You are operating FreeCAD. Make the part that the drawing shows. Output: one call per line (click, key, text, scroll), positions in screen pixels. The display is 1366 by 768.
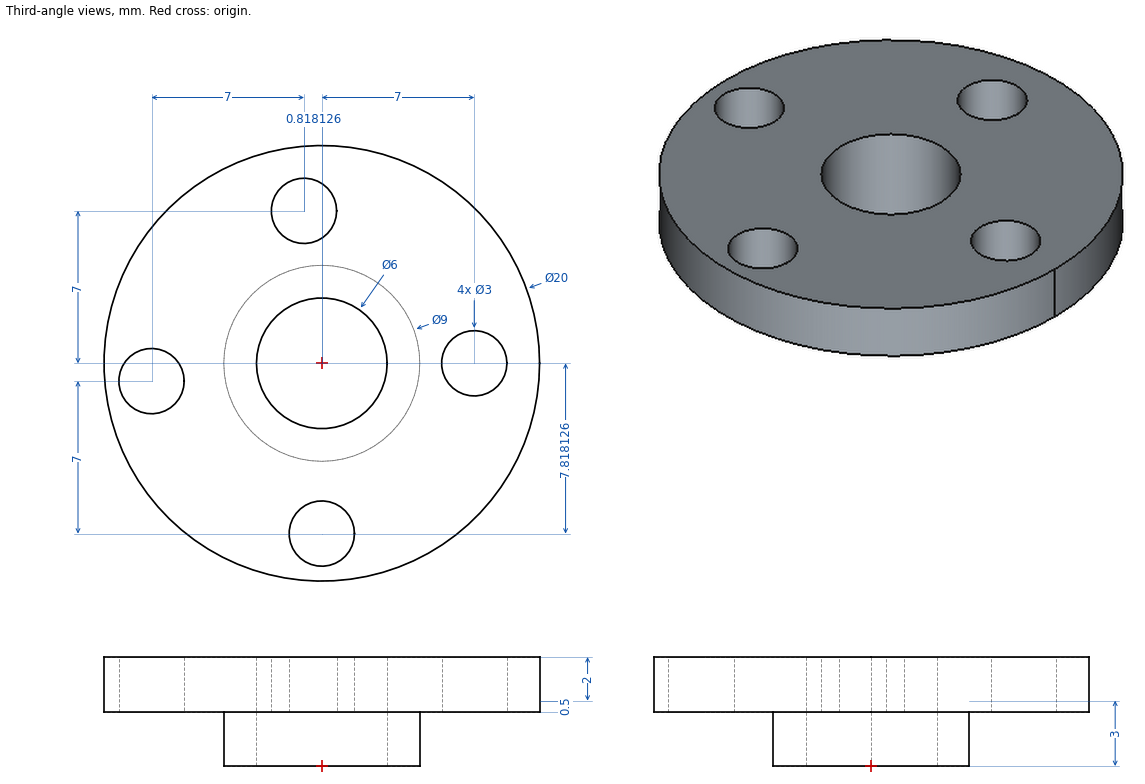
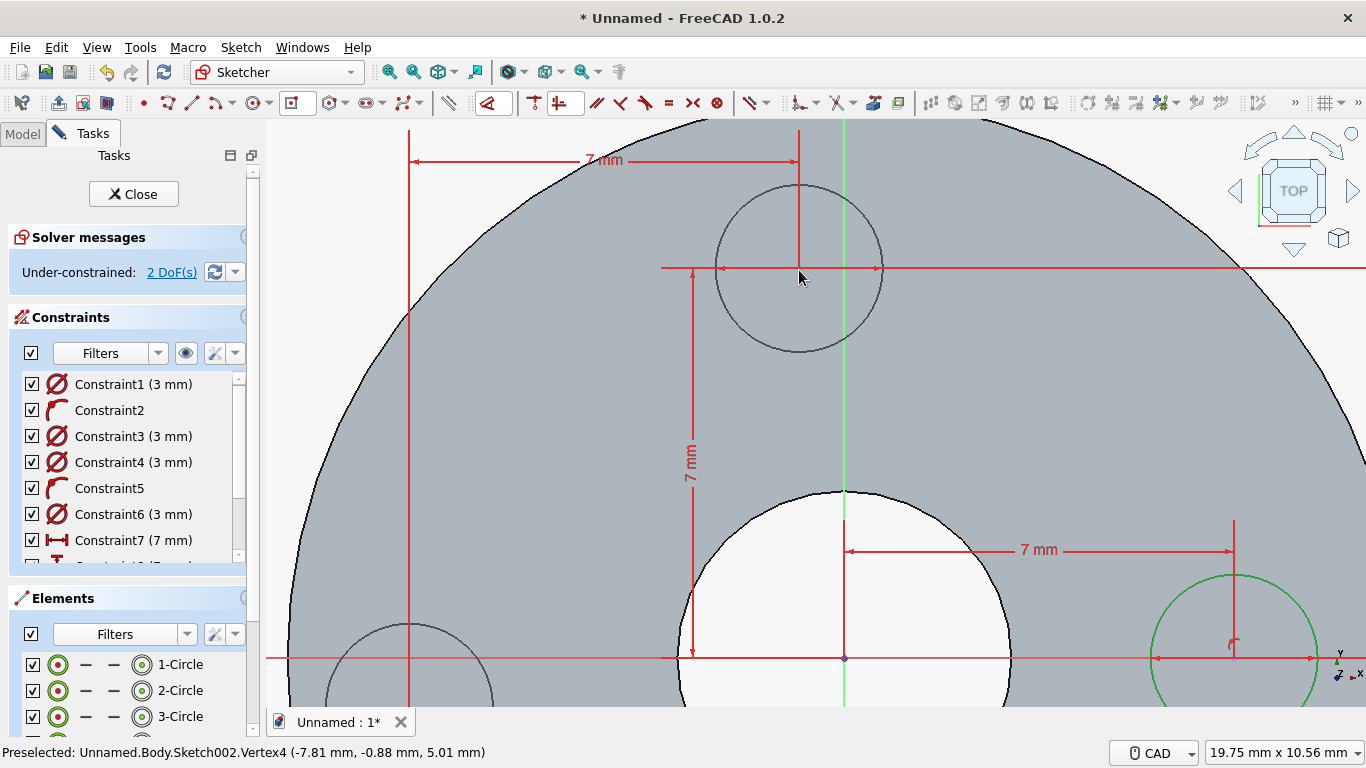
click(799, 268)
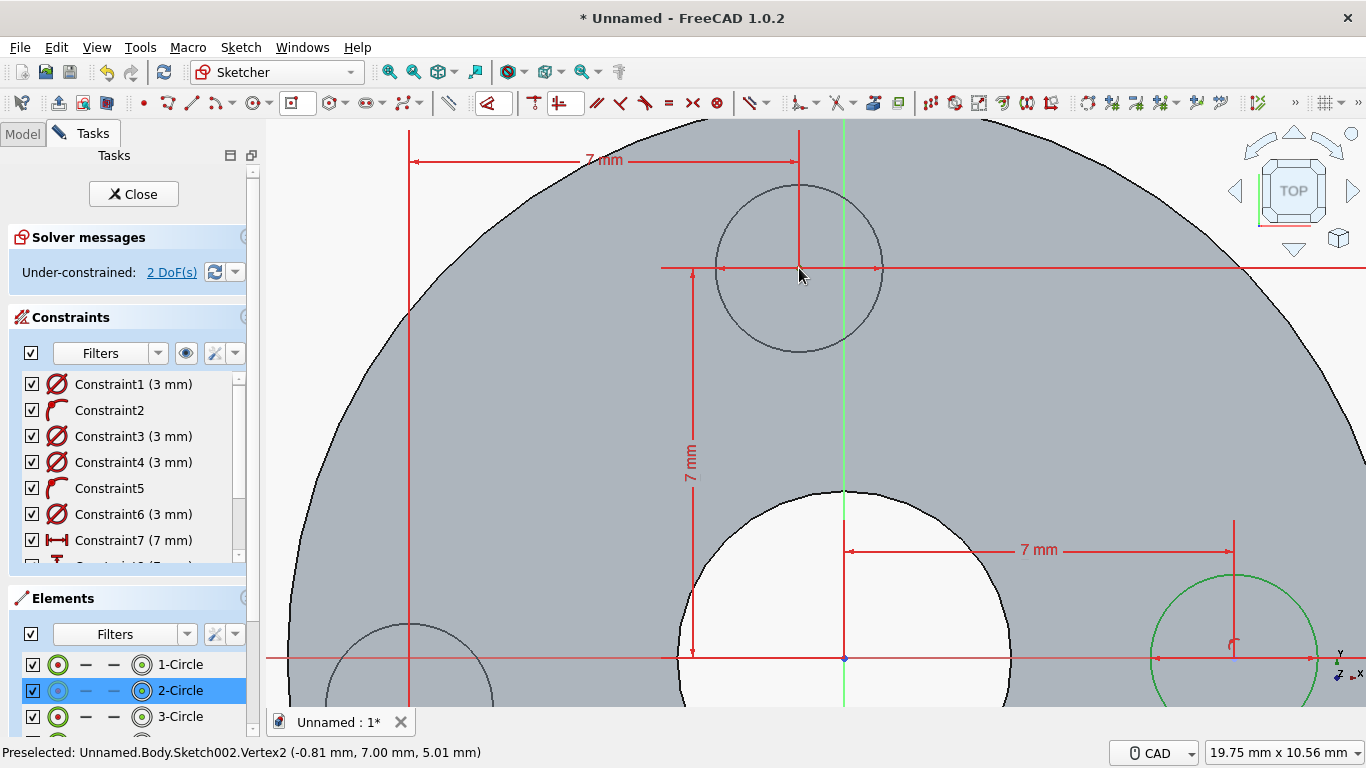
key(l)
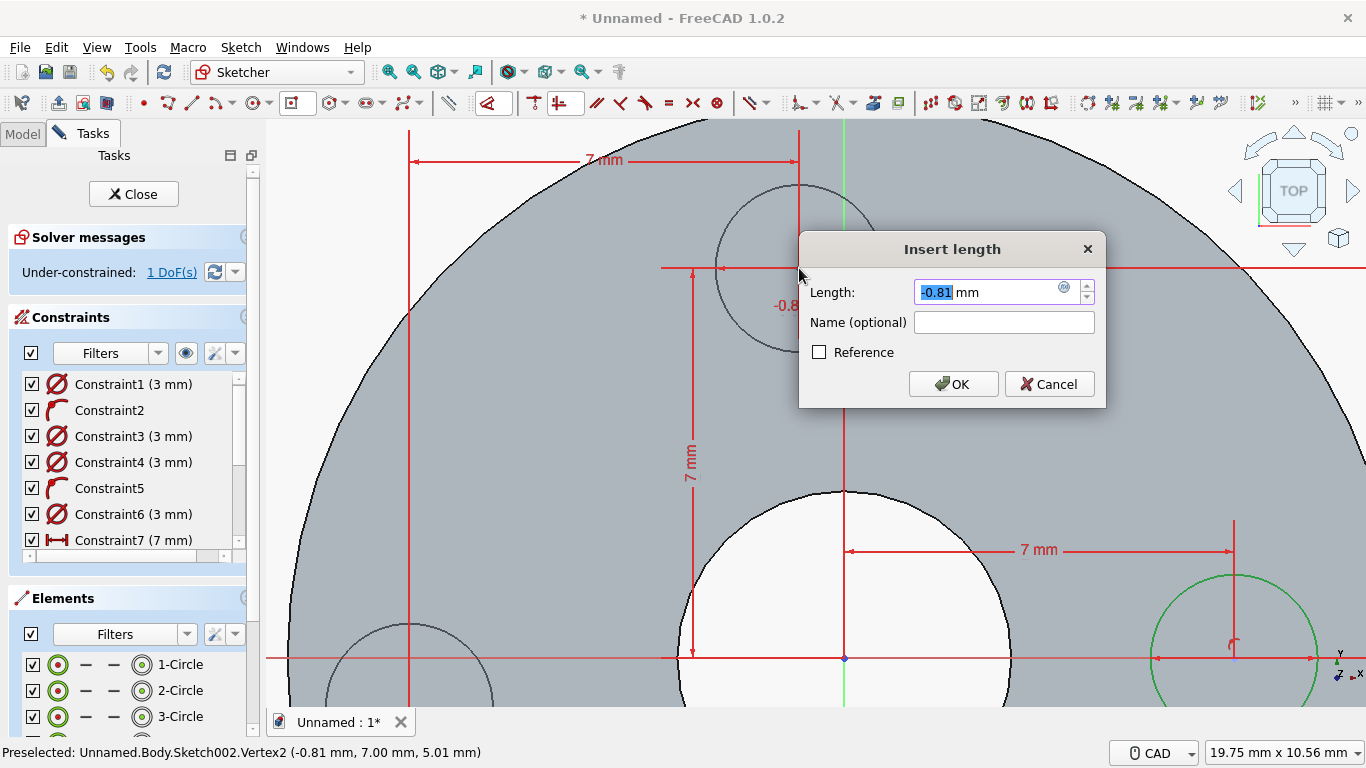
text(-0.818126)
key(Return)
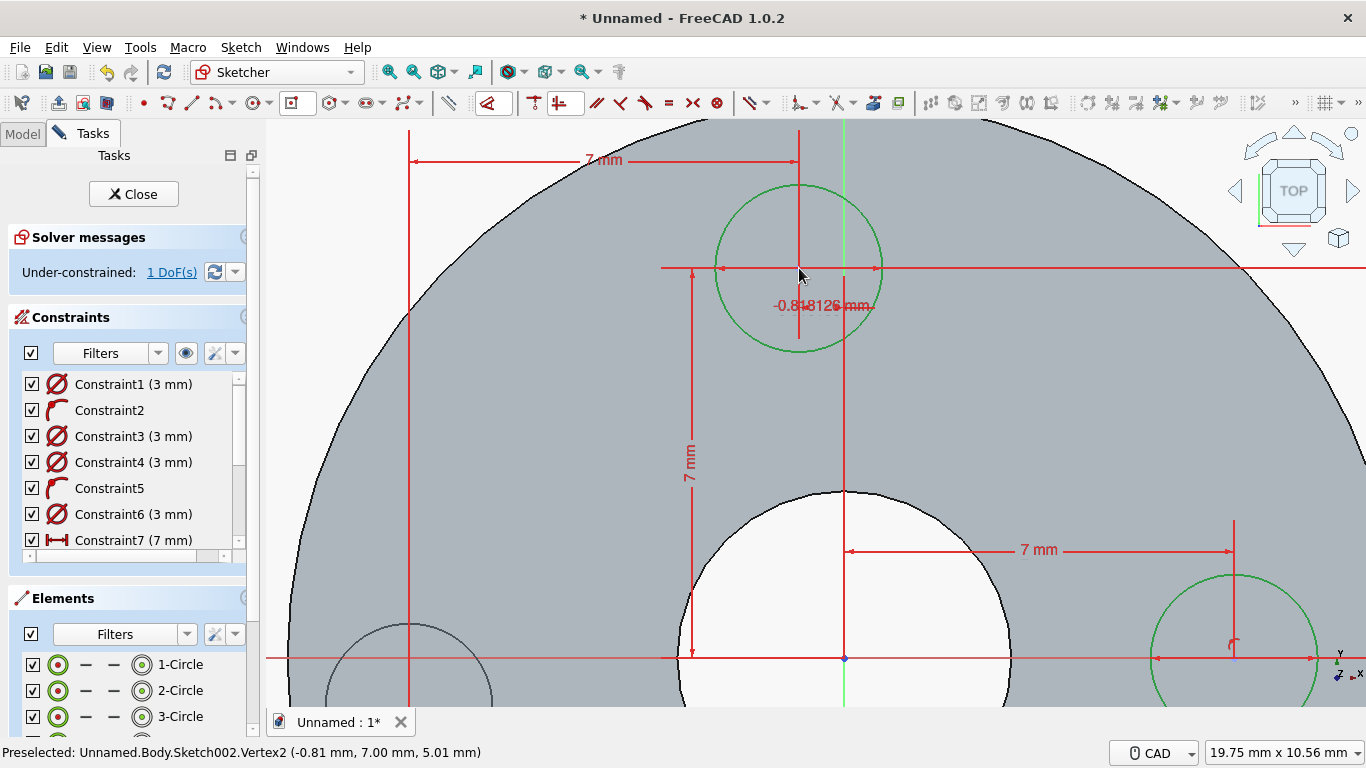
scroll(704, 257, down, 5)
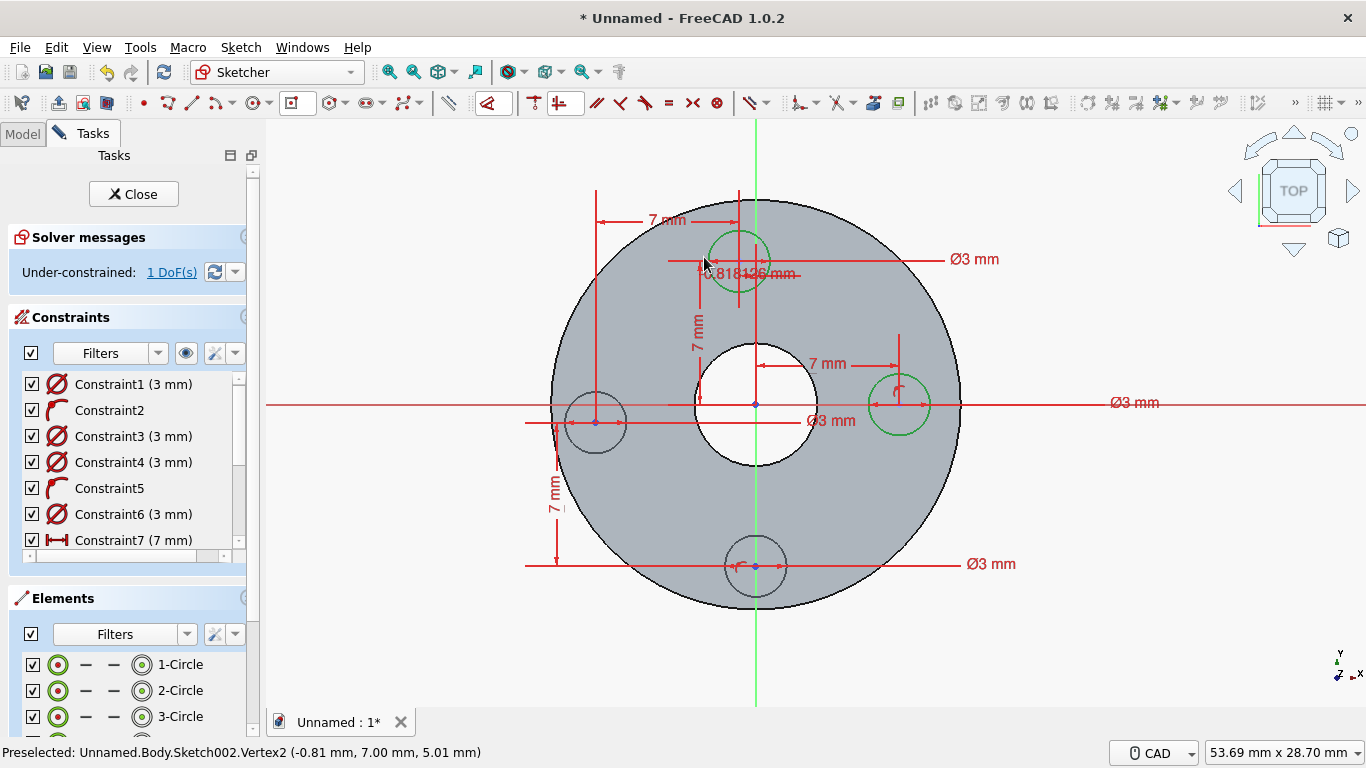
click(756, 566)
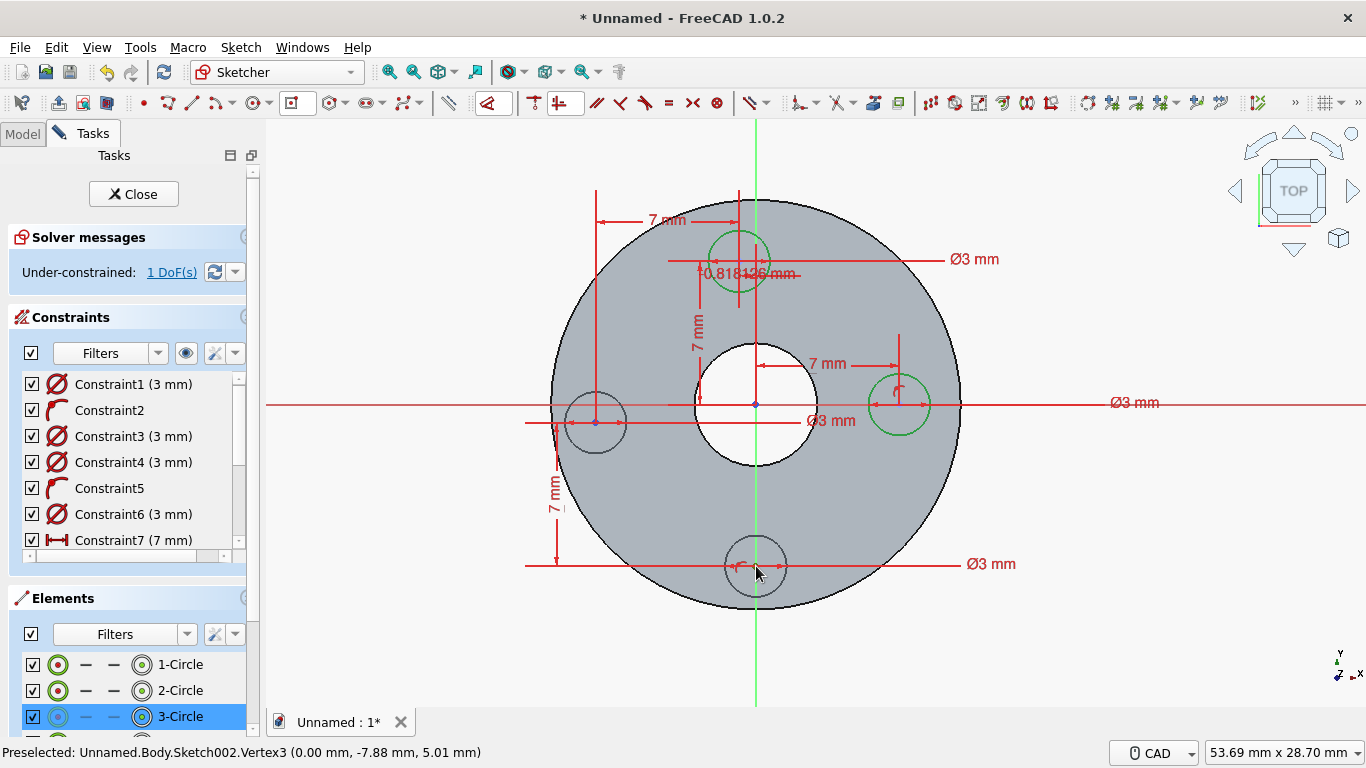
key(i)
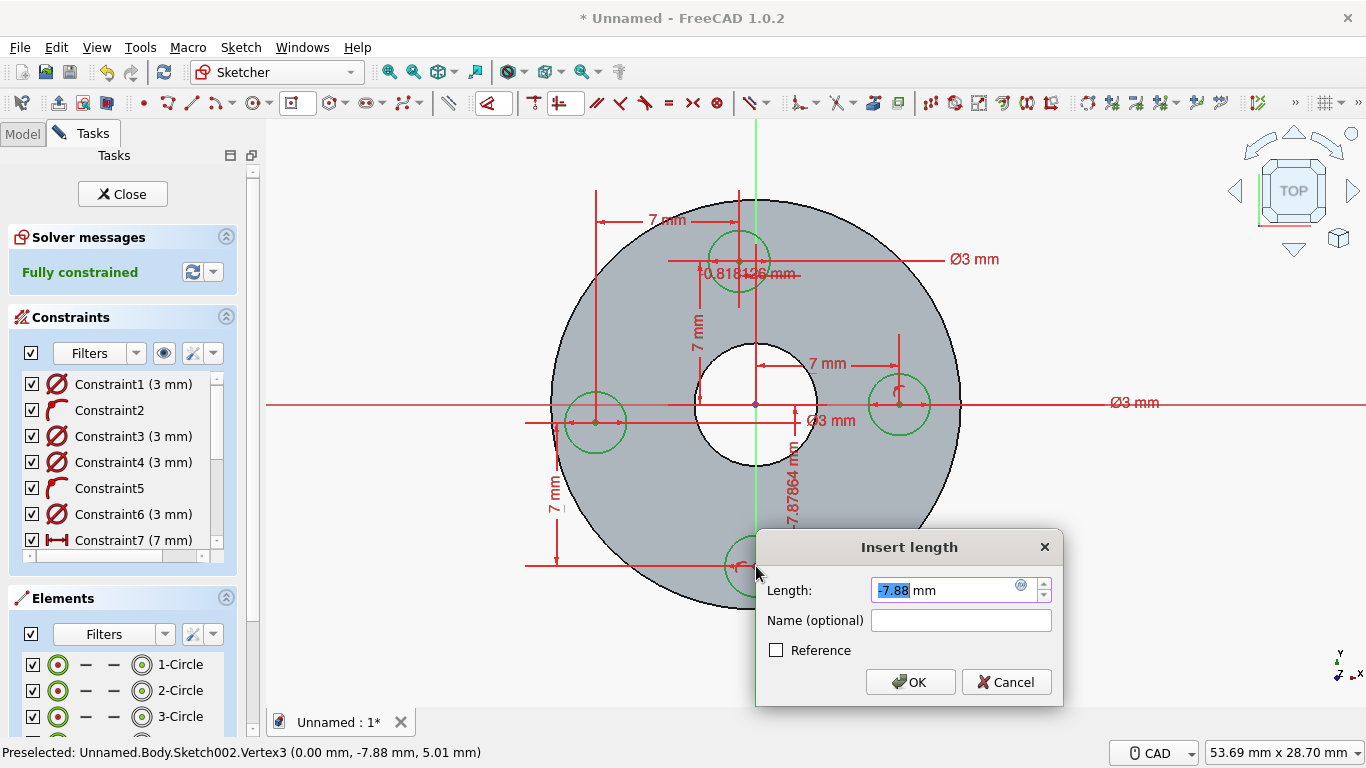
text(-7.818126)
key(Return)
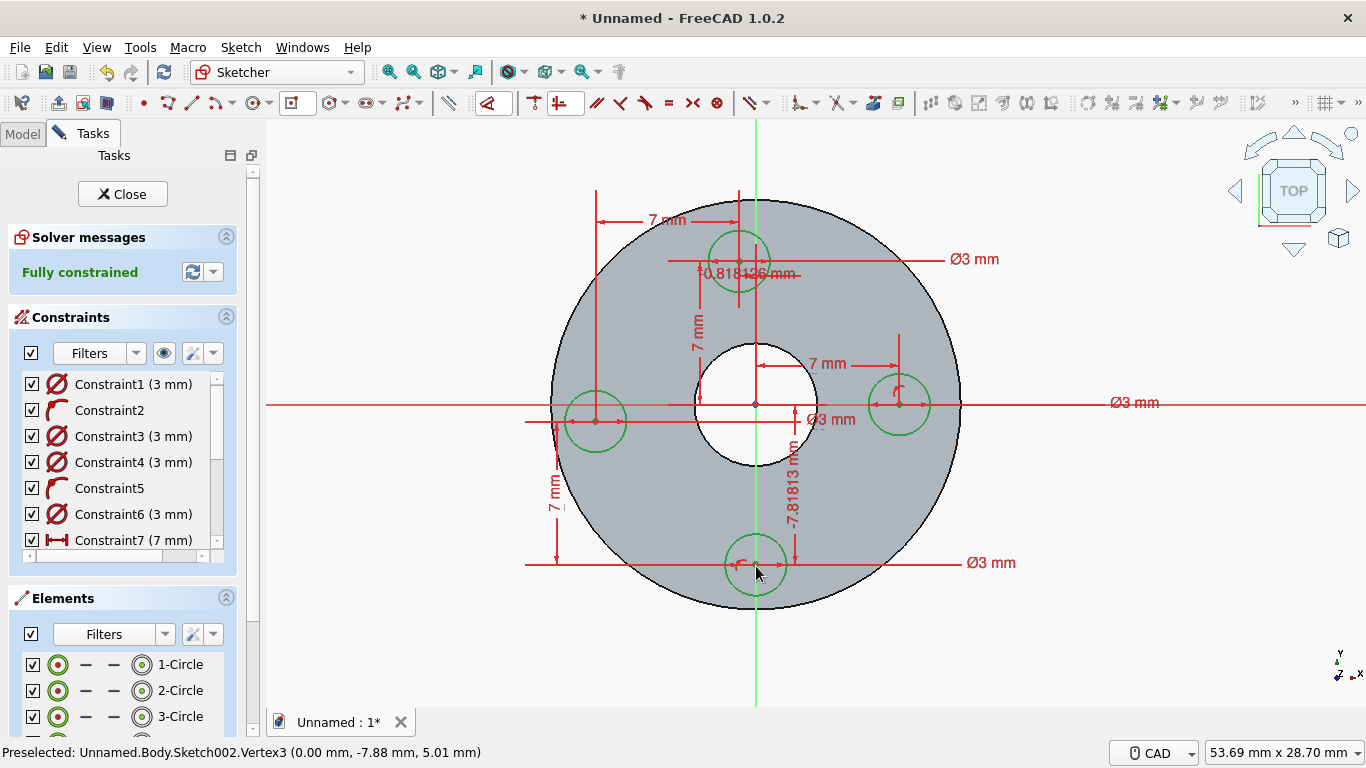
click(123, 194)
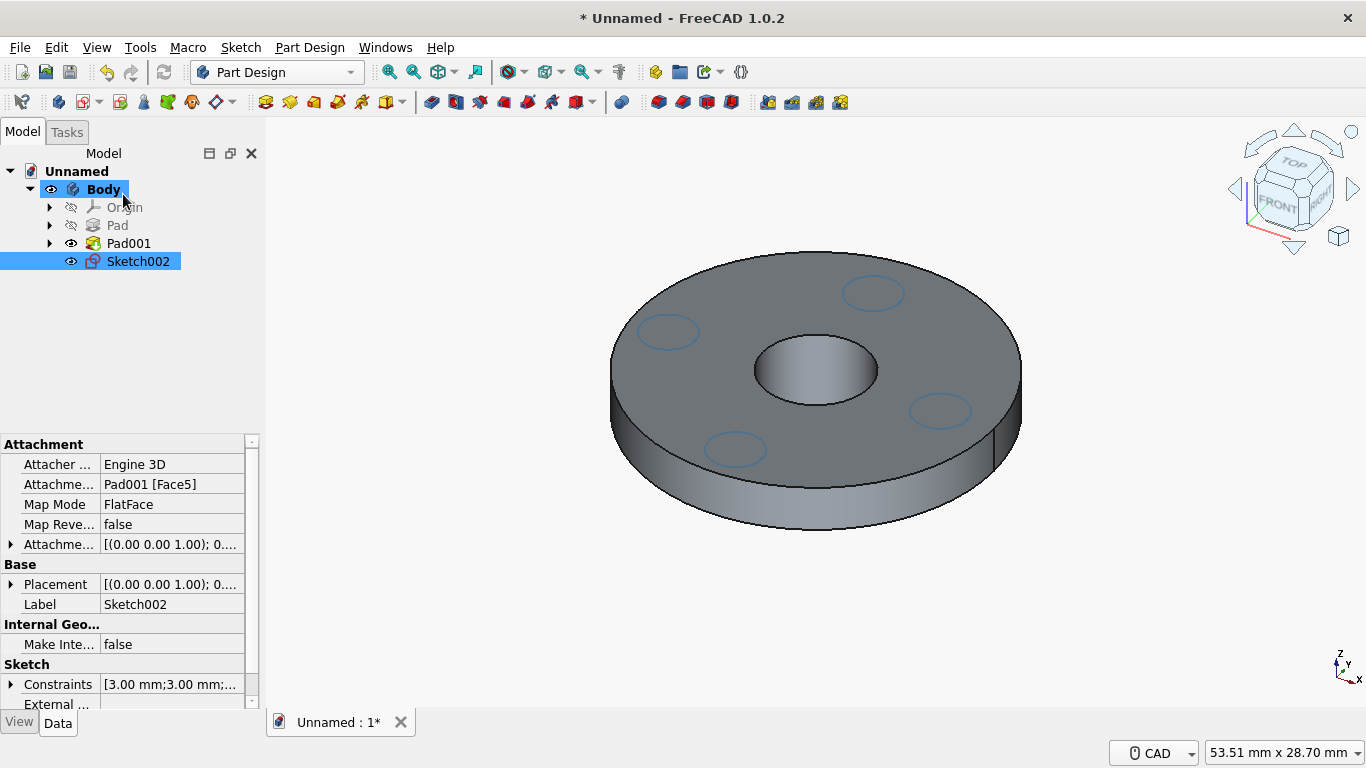
click(432, 102)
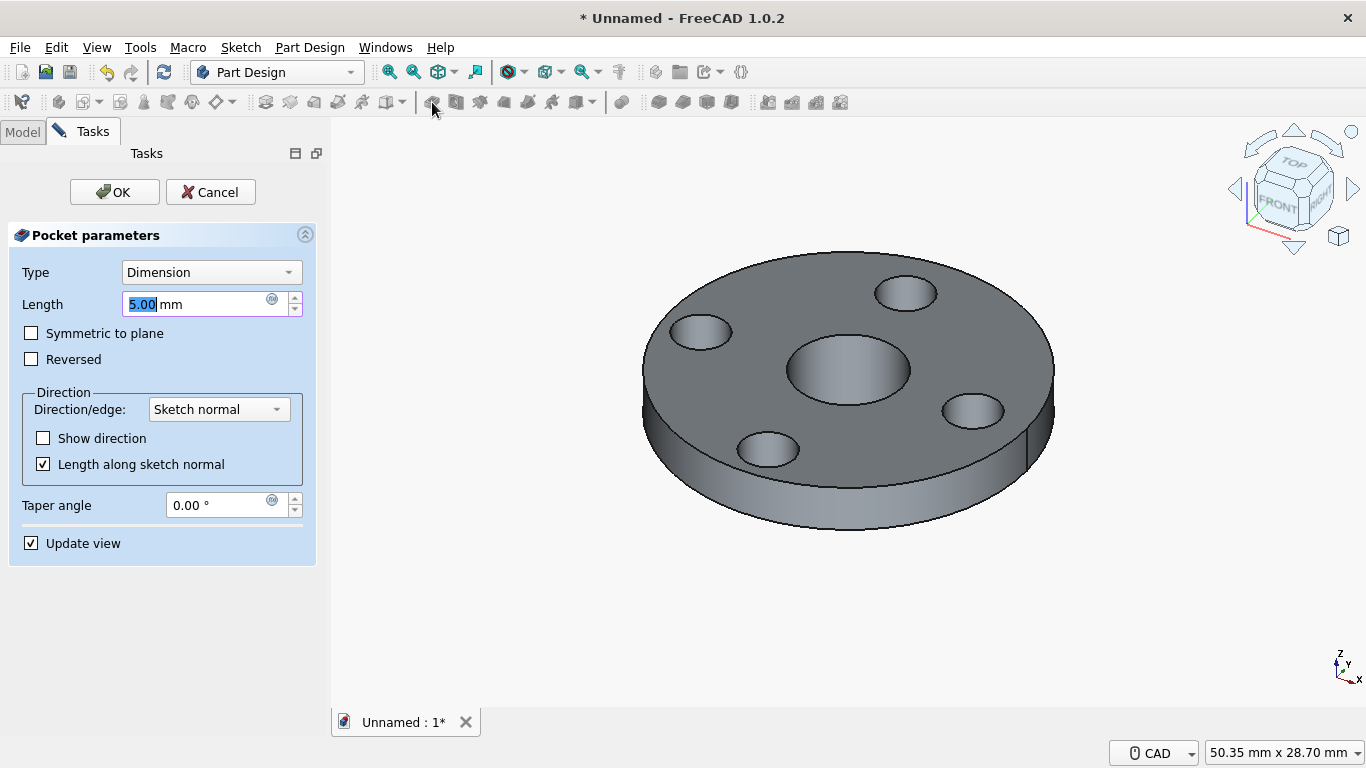
click(212, 272)